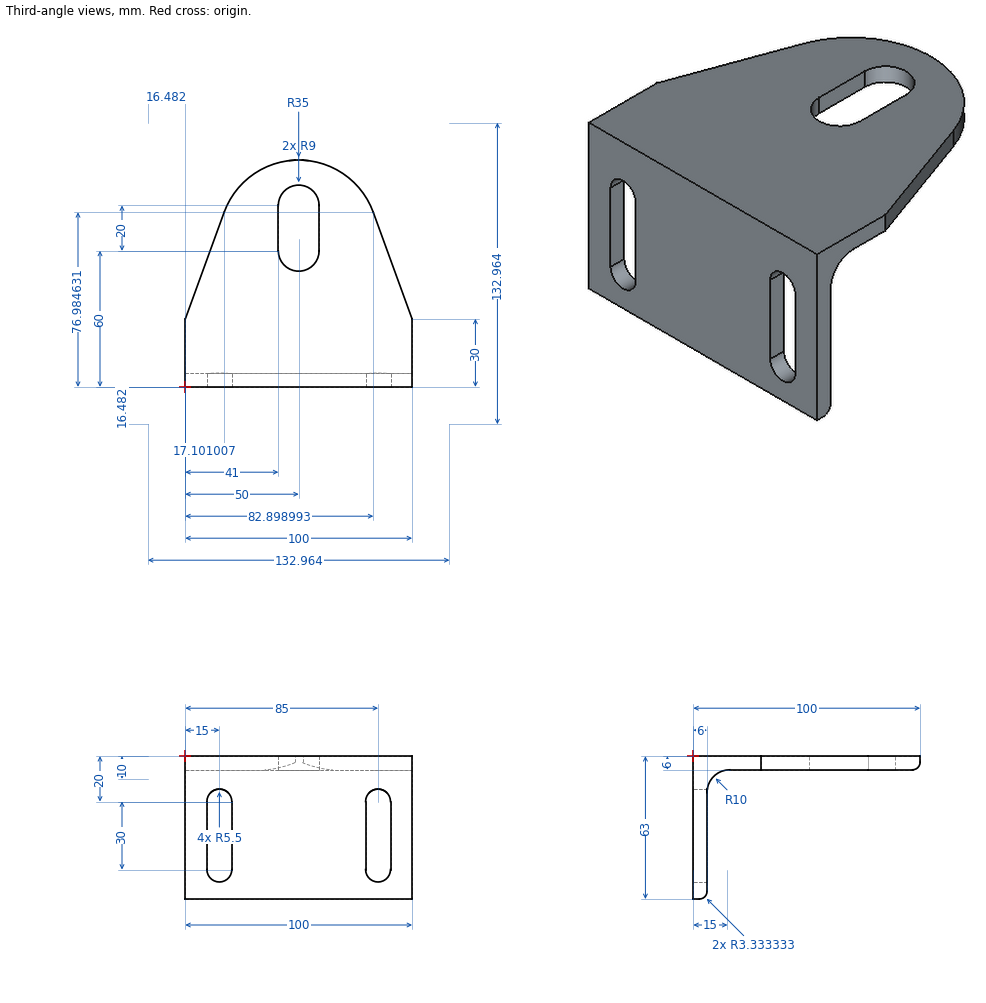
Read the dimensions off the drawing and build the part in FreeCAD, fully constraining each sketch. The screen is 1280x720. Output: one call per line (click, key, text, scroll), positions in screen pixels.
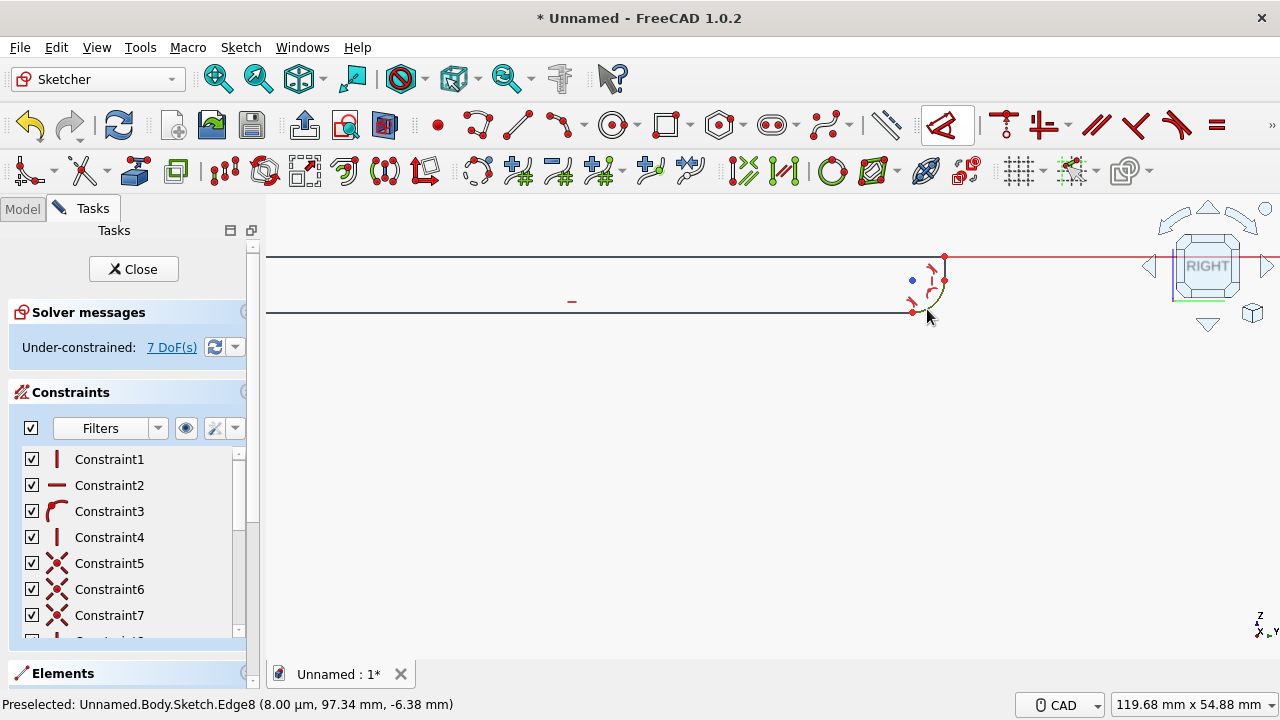
scroll(927, 308, down, 3)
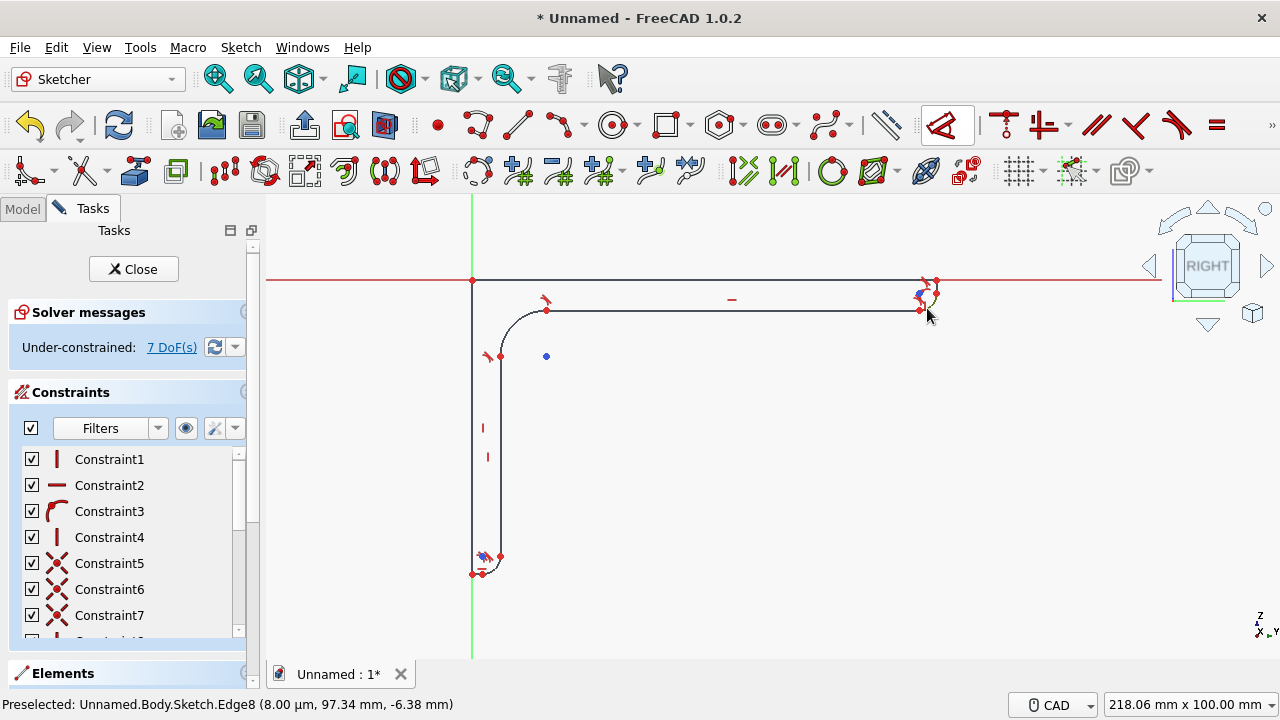
scroll(491, 572, up, 3)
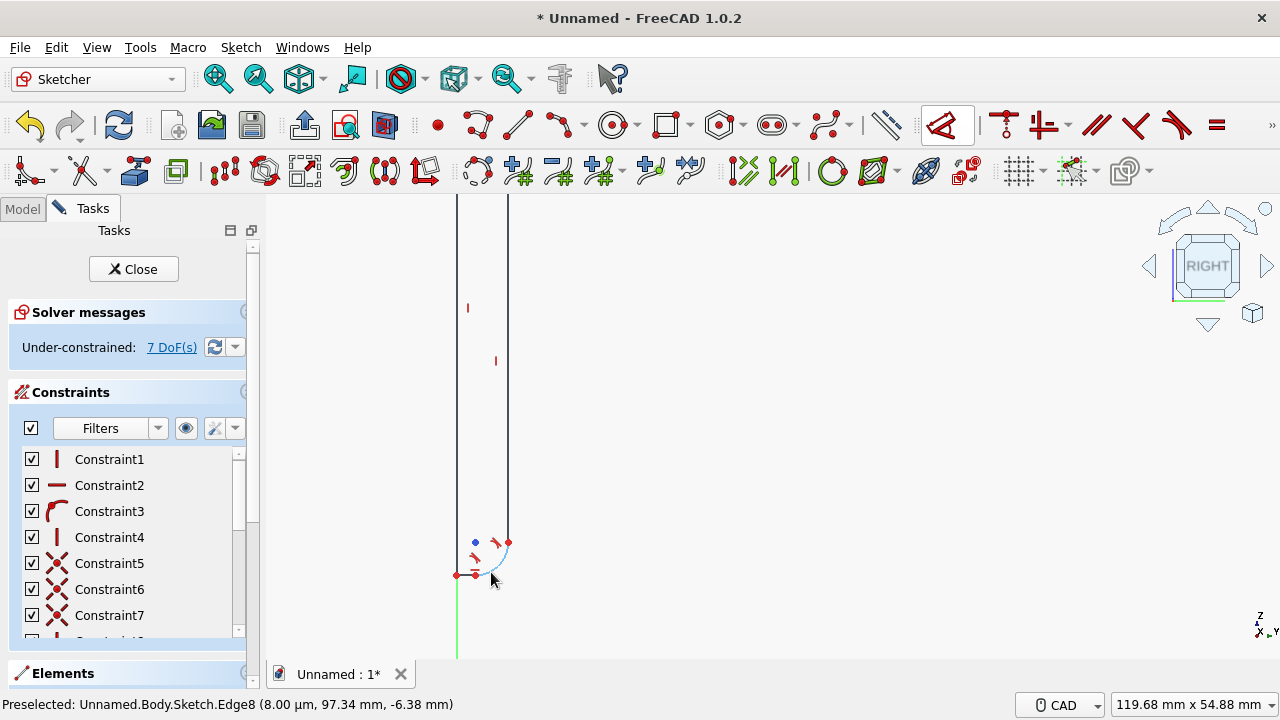
click(490, 572)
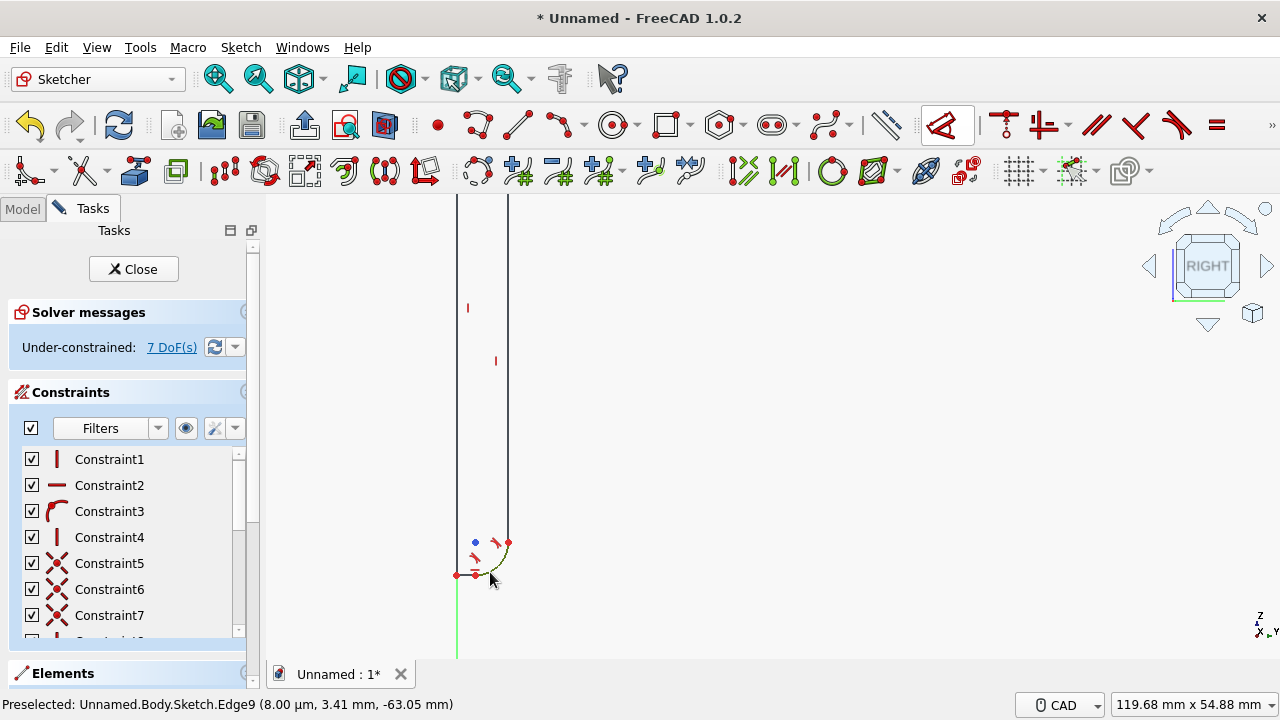
click(1218, 126)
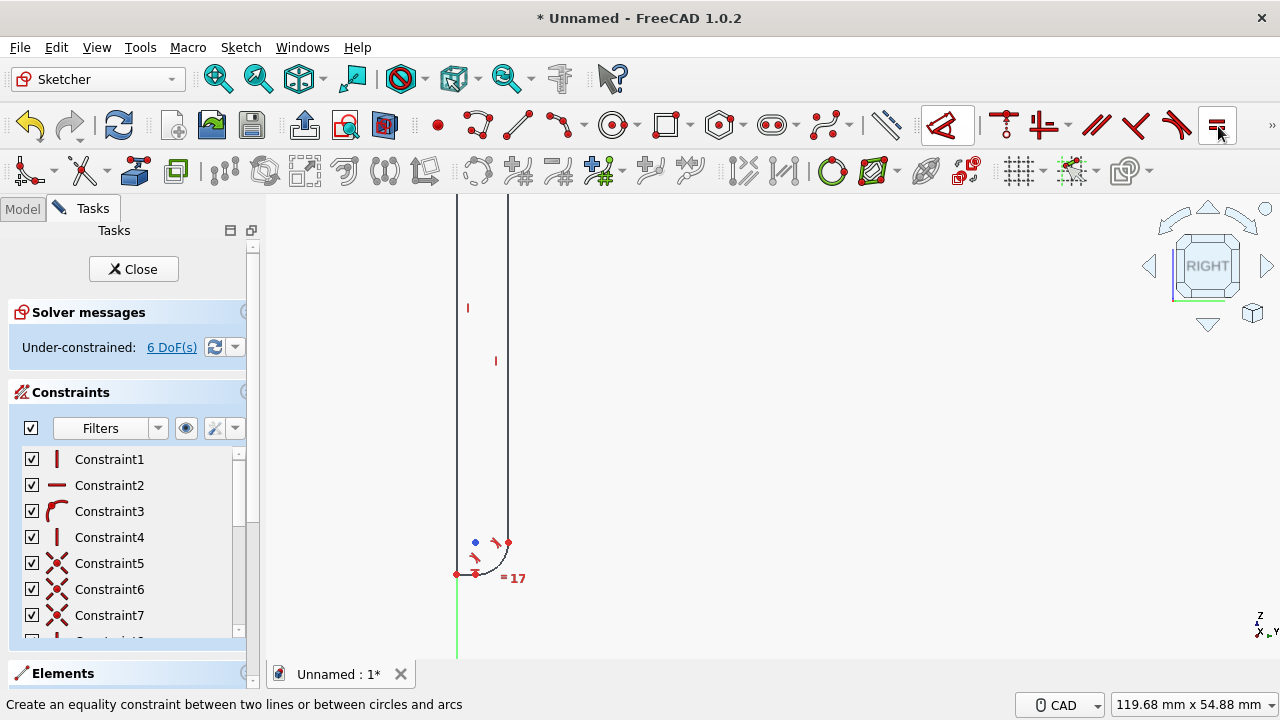
scroll(491, 573, down, 3)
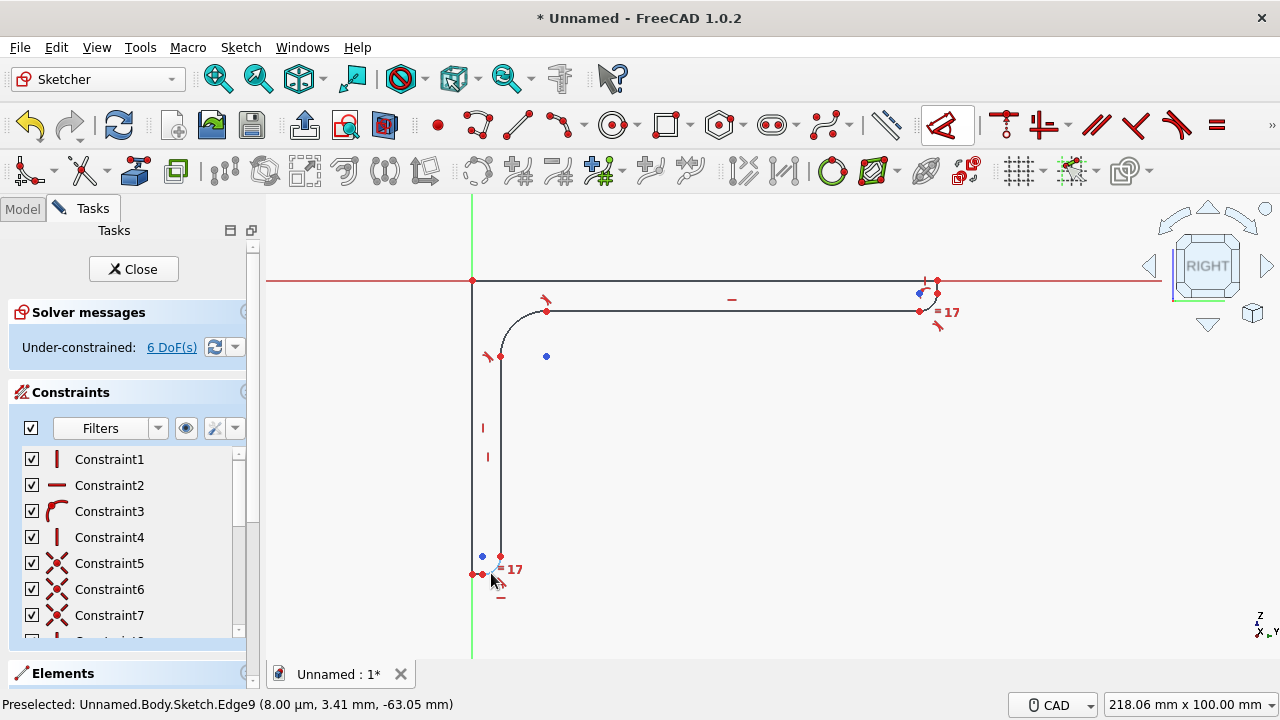
click(526, 316)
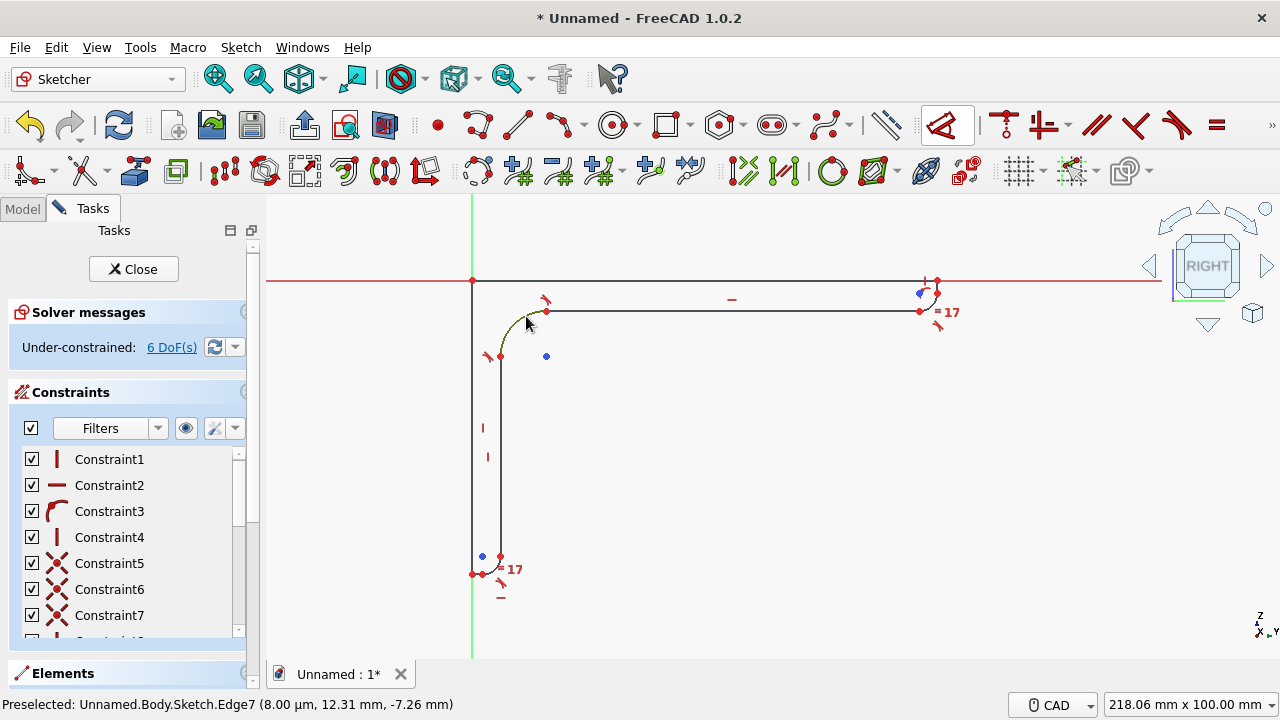
key(k)
key(r)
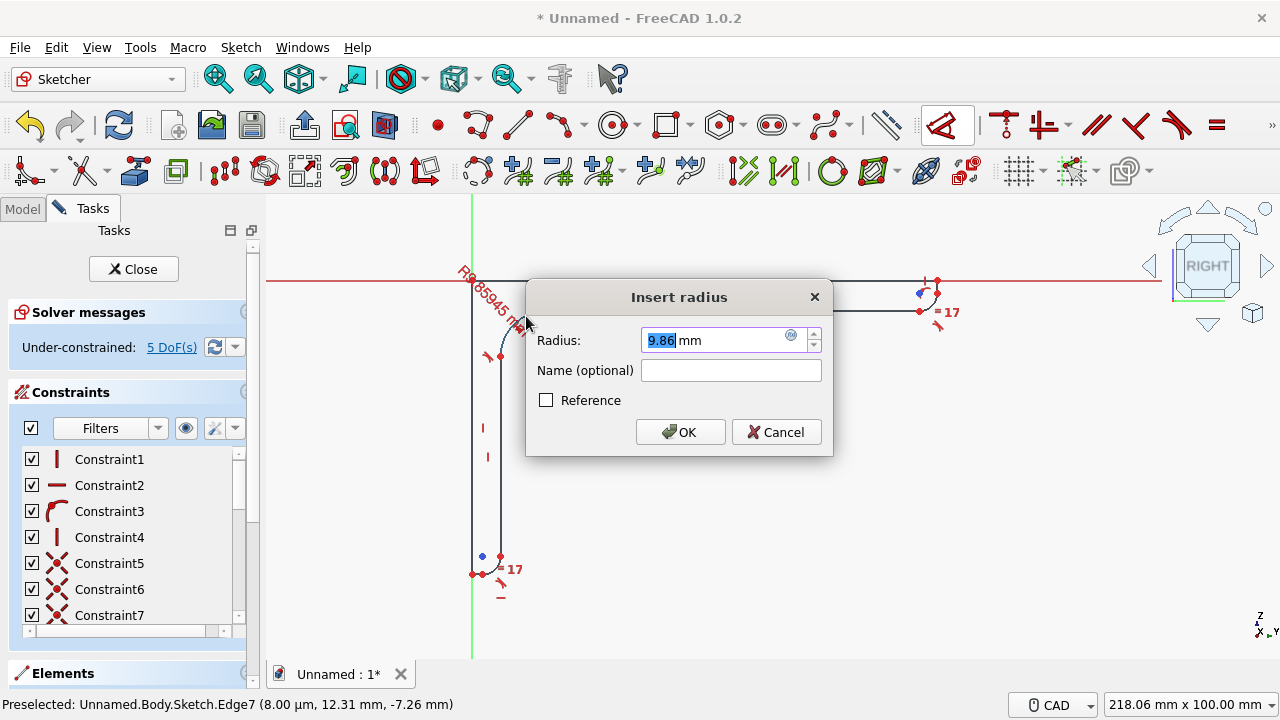
text(10)
key(Return)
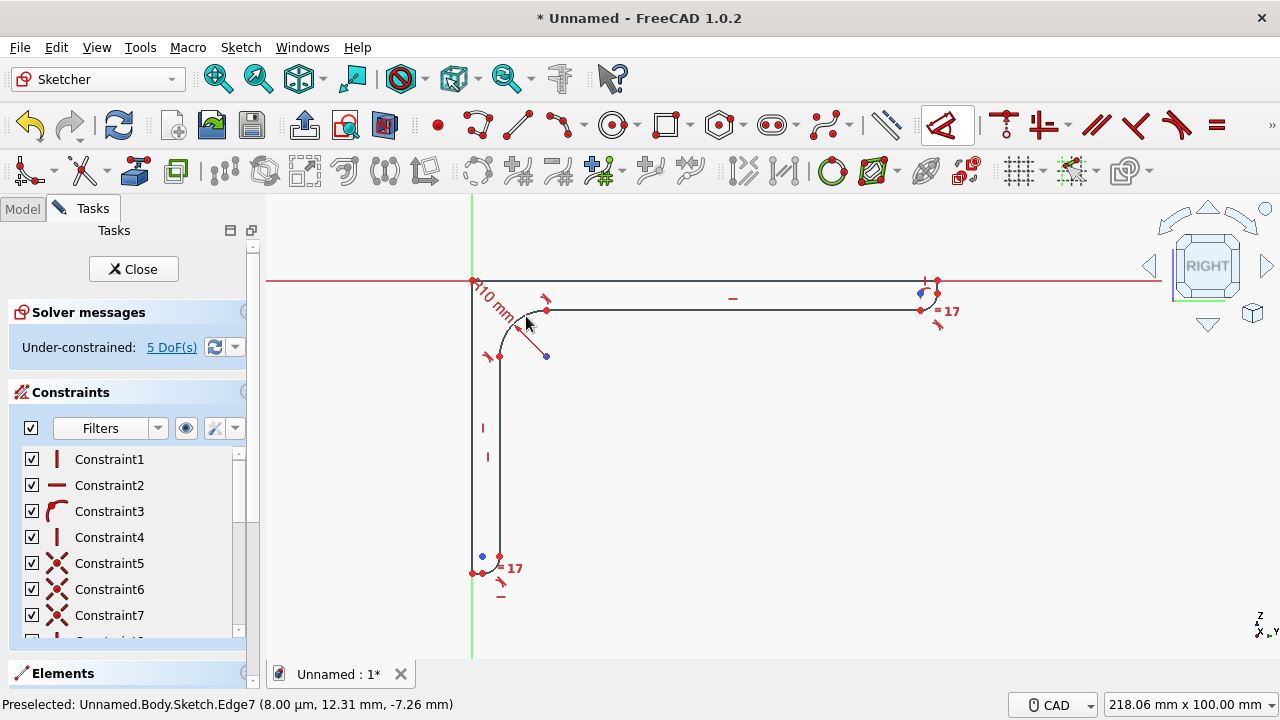
scroll(932, 305, up, 5)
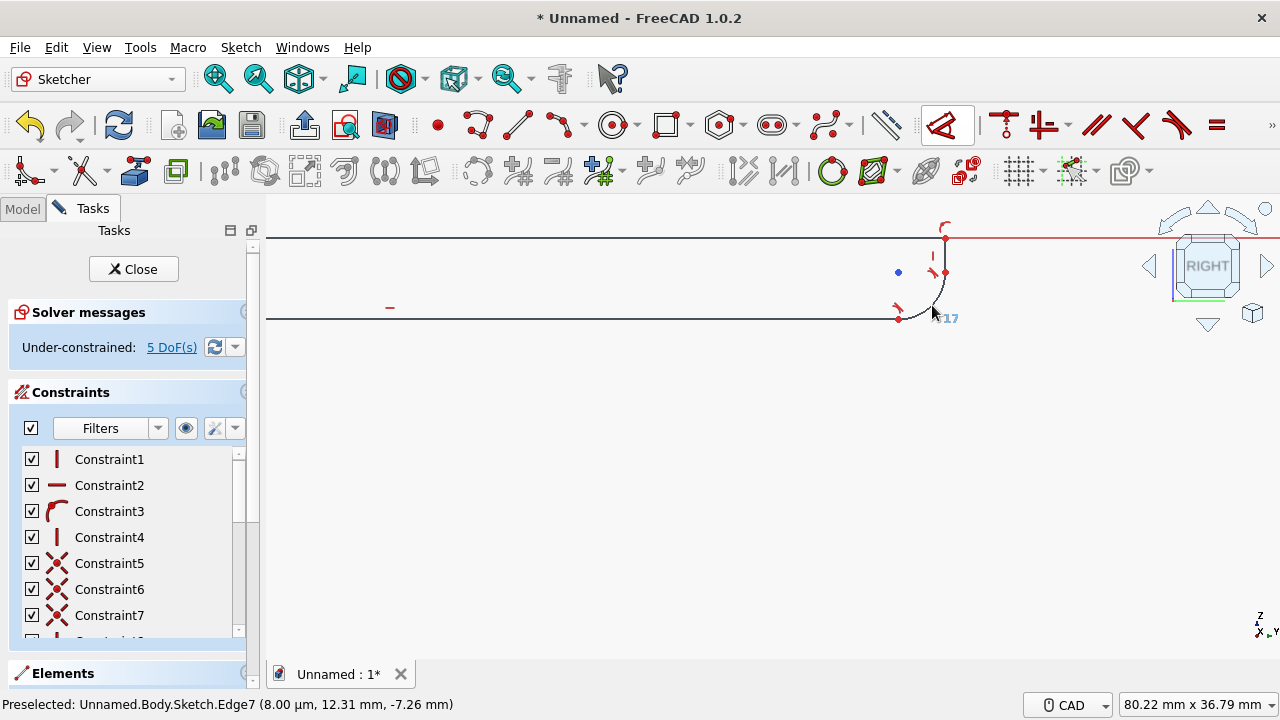
click(931, 306)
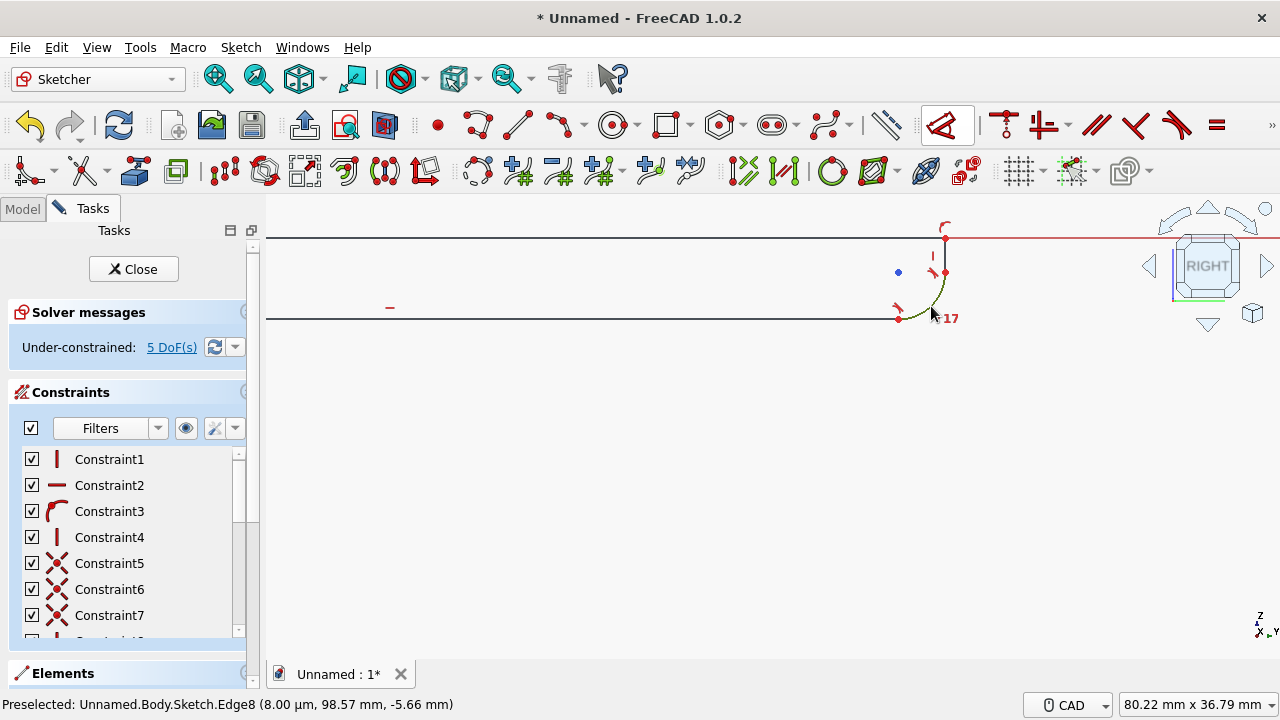
key(k)
key(r)